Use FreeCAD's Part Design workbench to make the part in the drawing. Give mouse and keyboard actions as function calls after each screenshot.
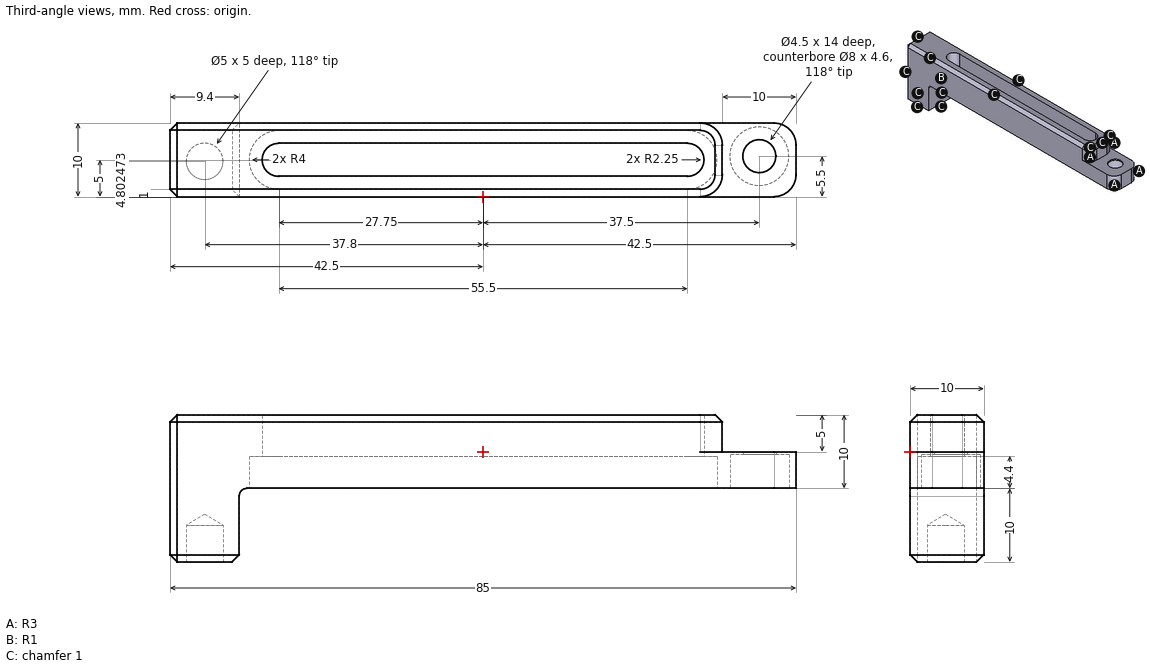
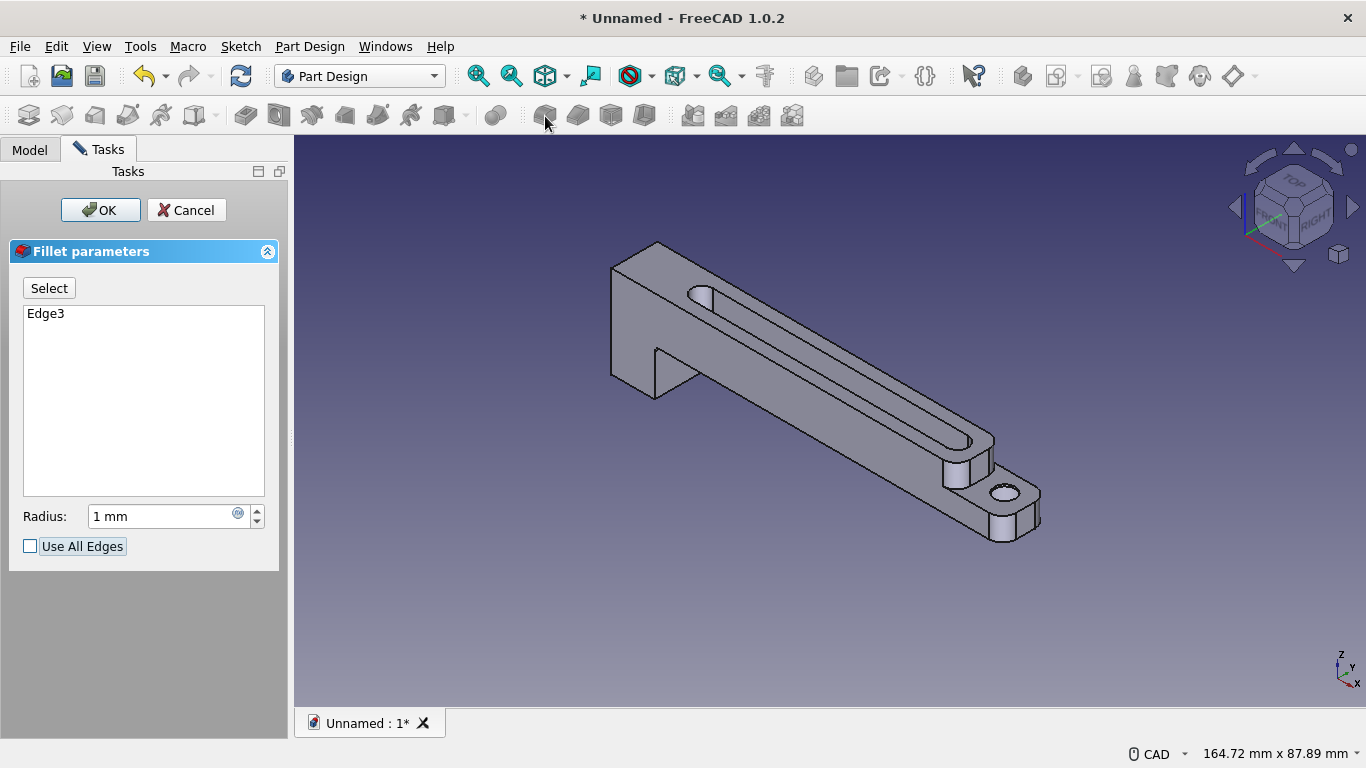
click(101, 210)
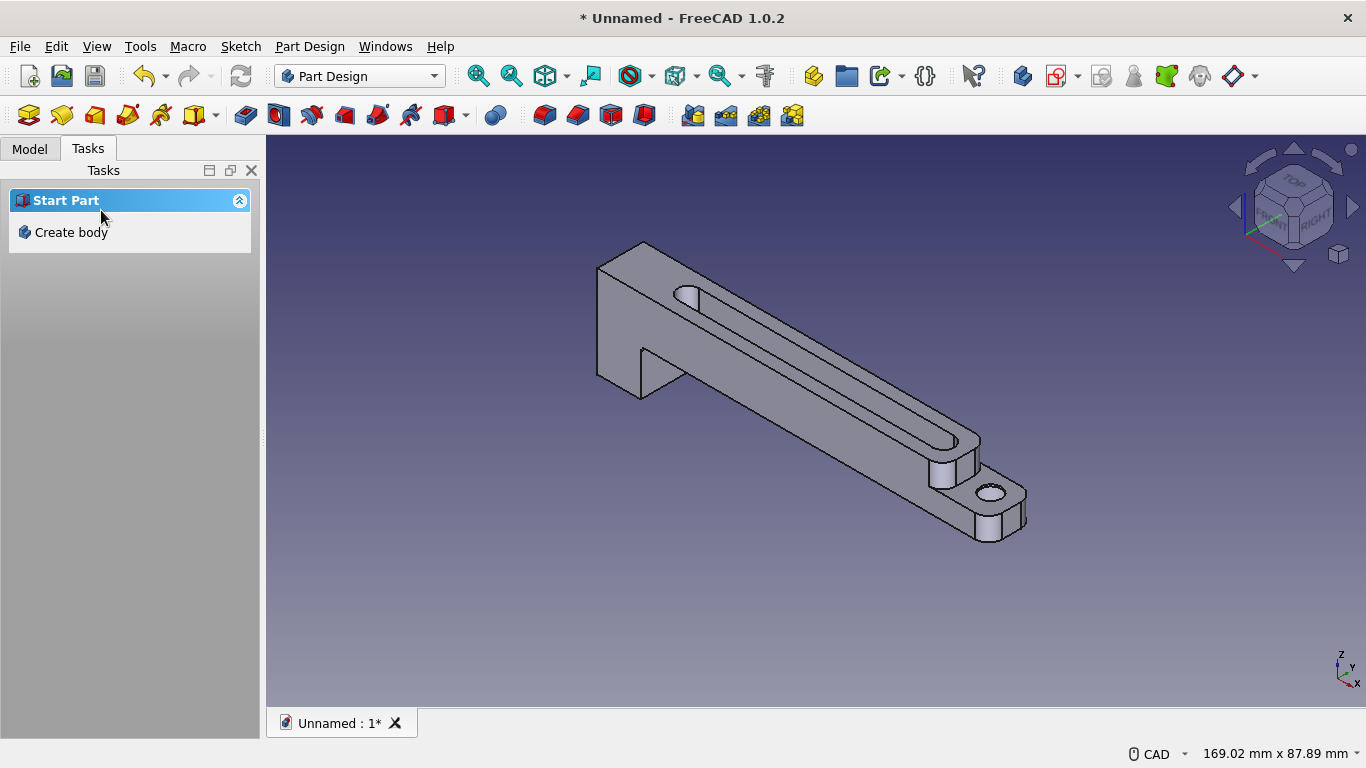
click(763, 363)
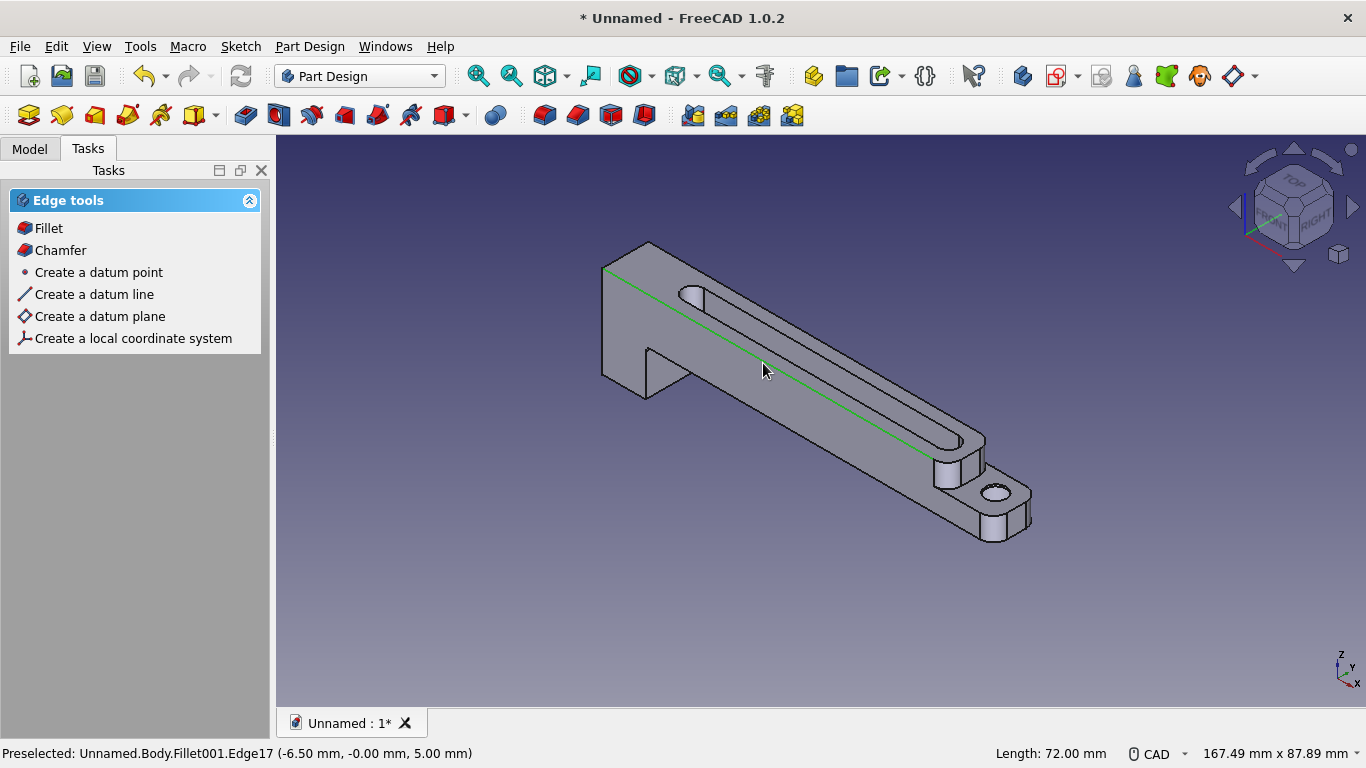
click(971, 453, ctrl)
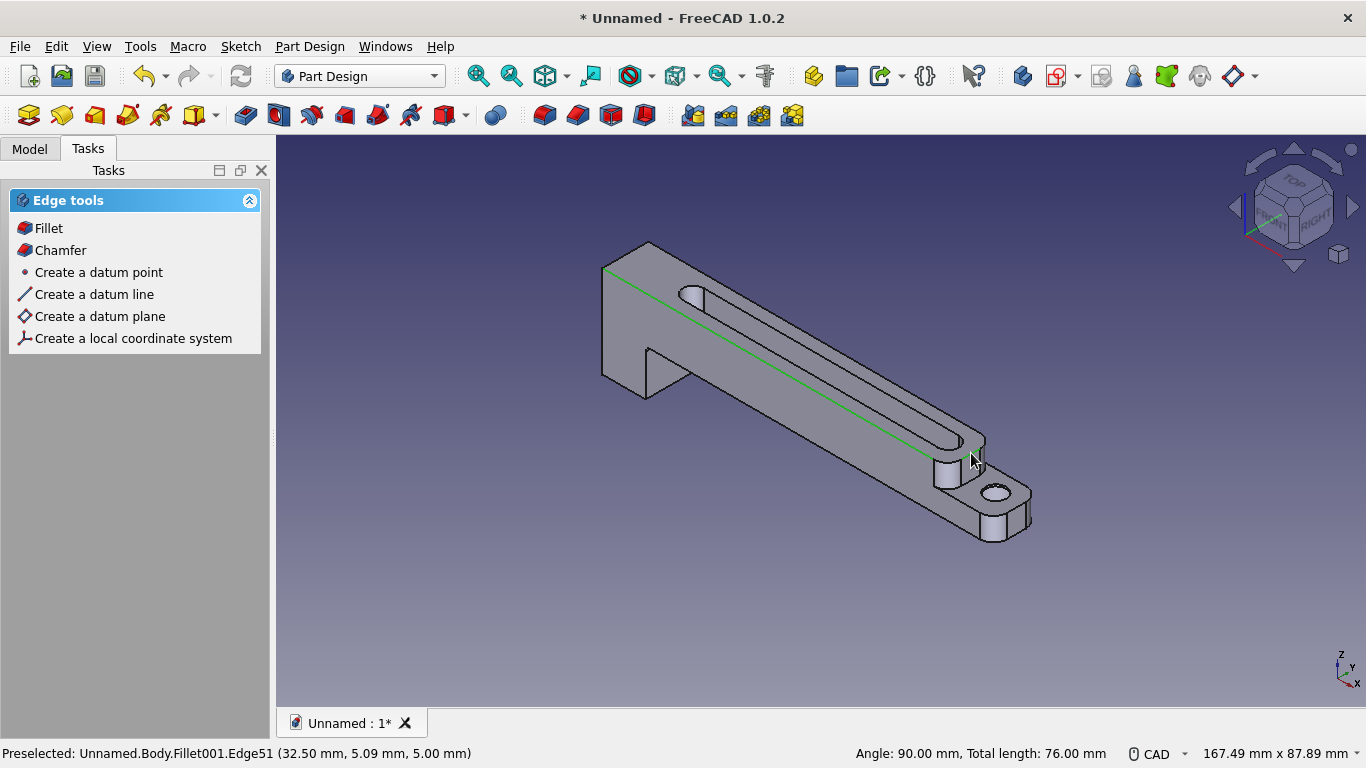
click(985, 440, ctrl)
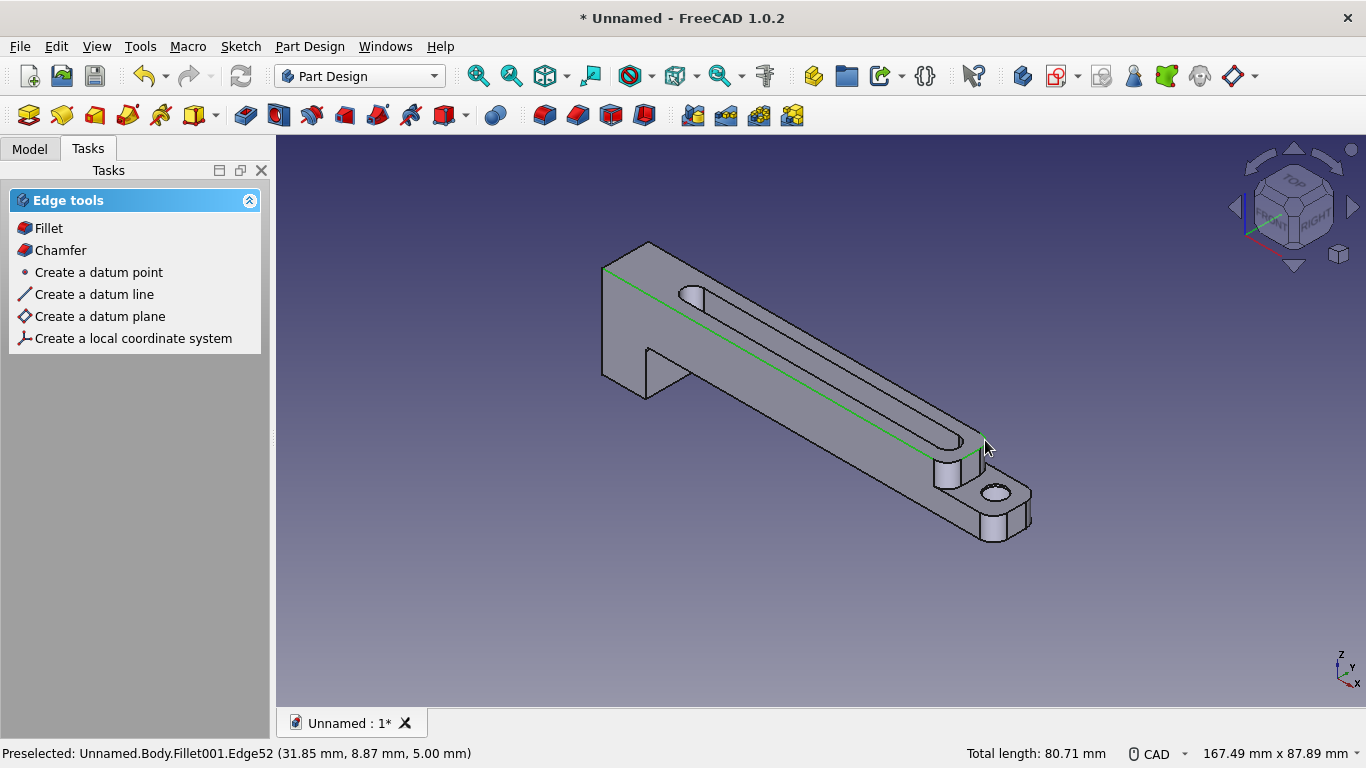
click(948, 462, ctrl)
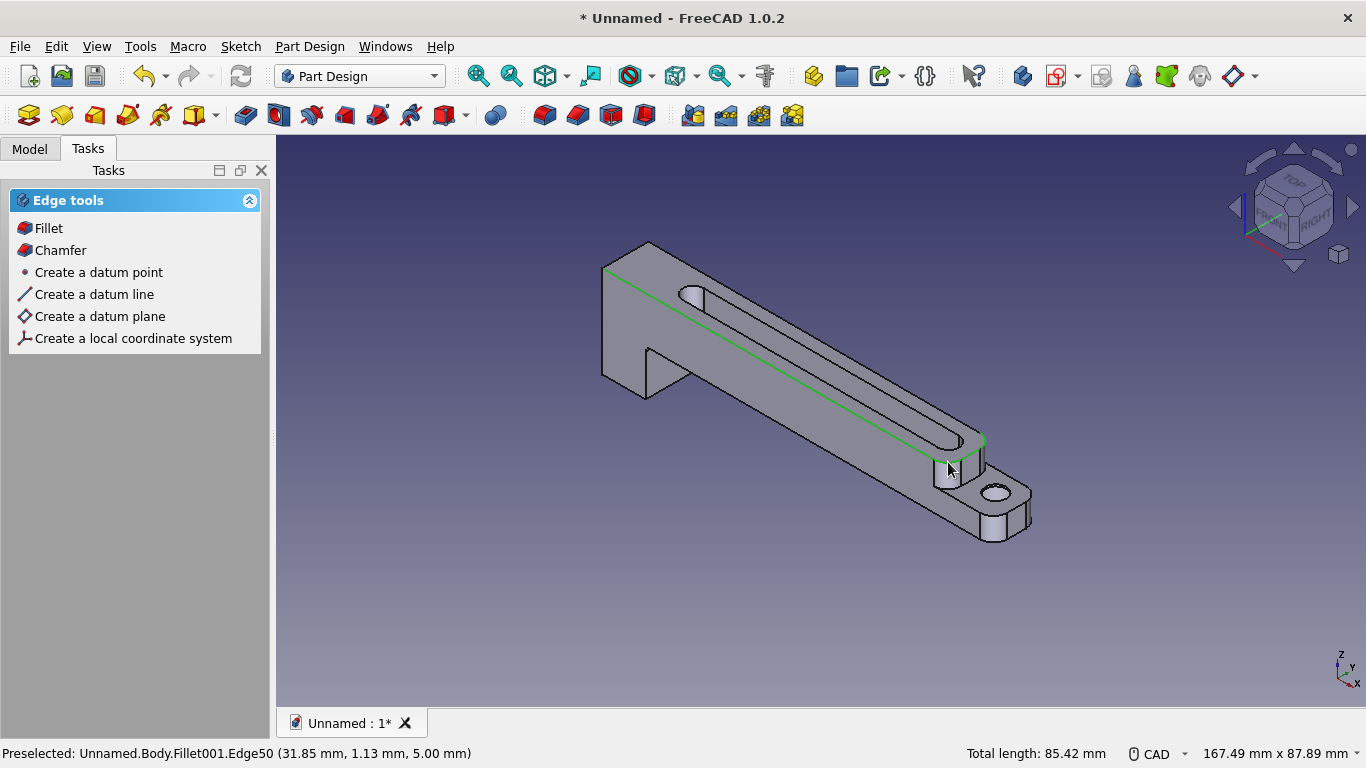
key(2)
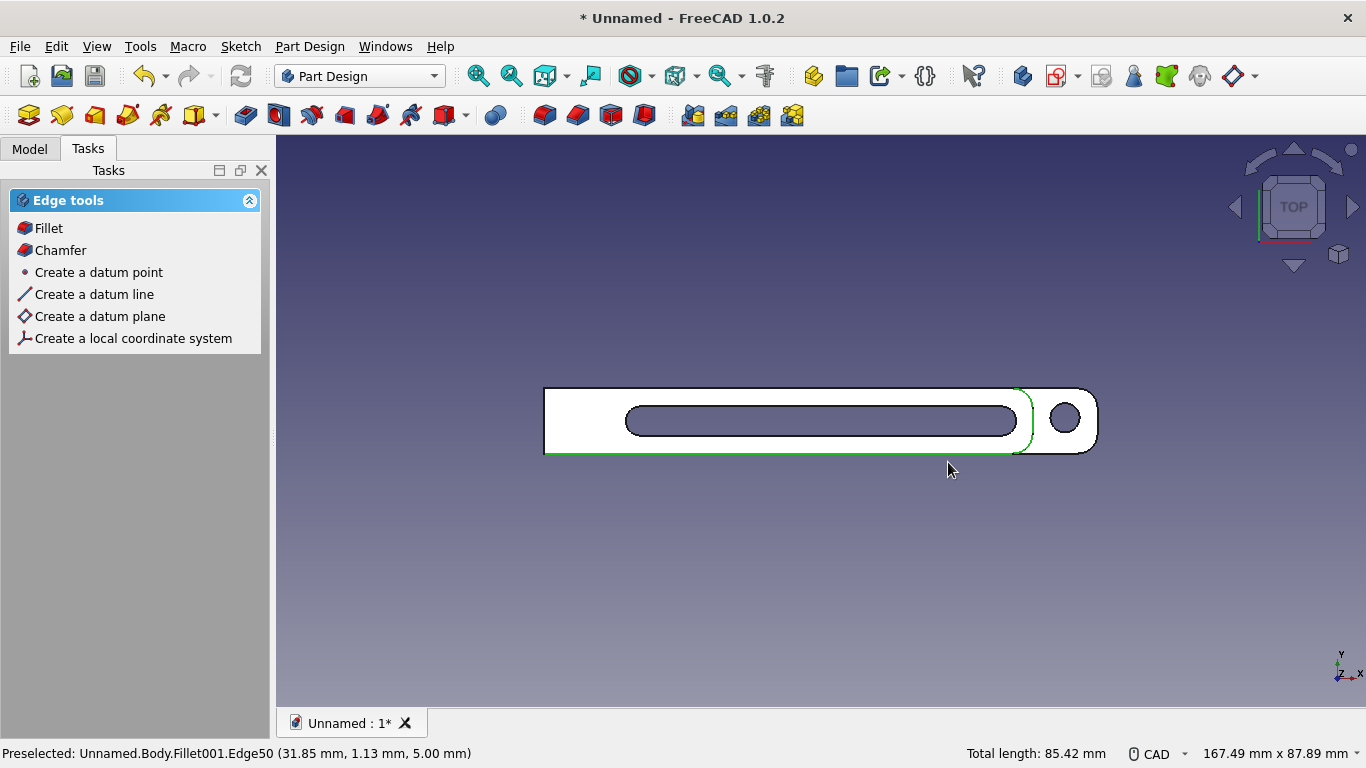
click(779, 387, ctrl)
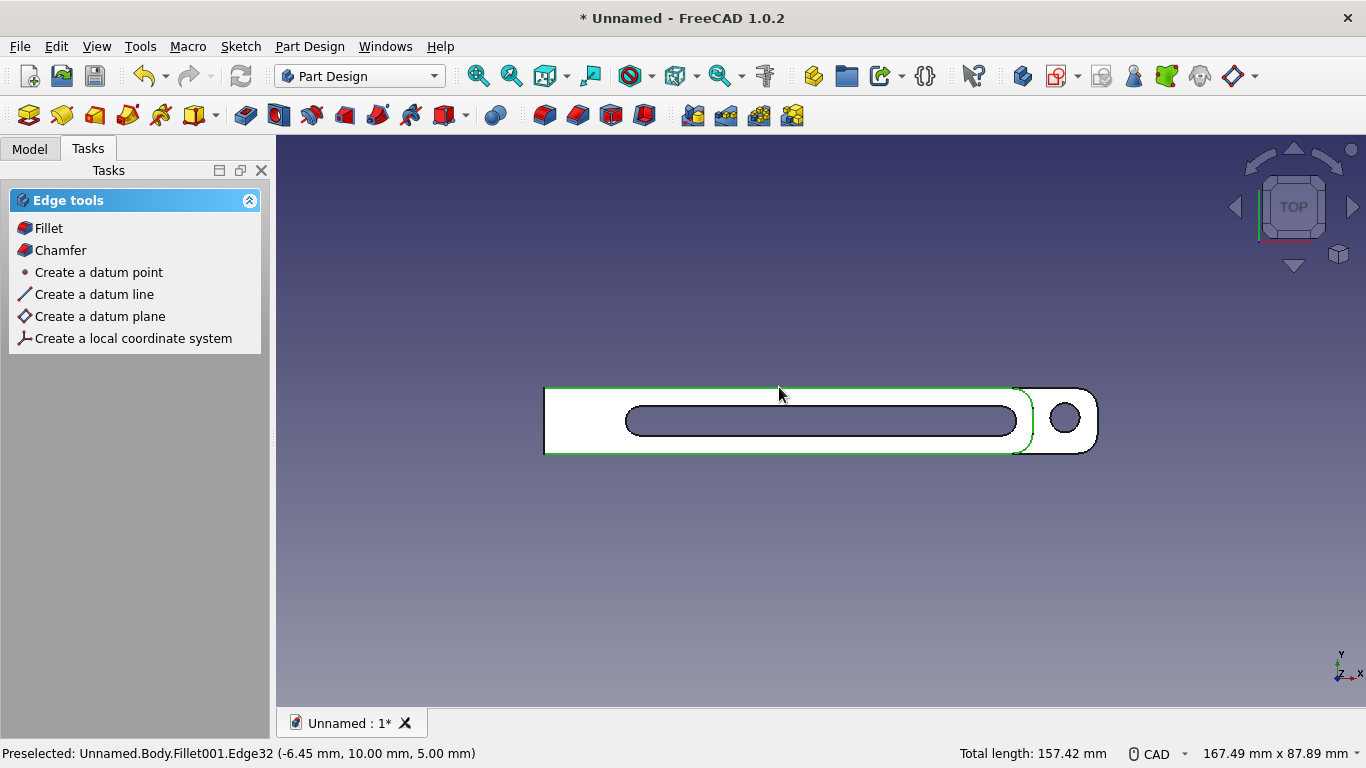
key(0)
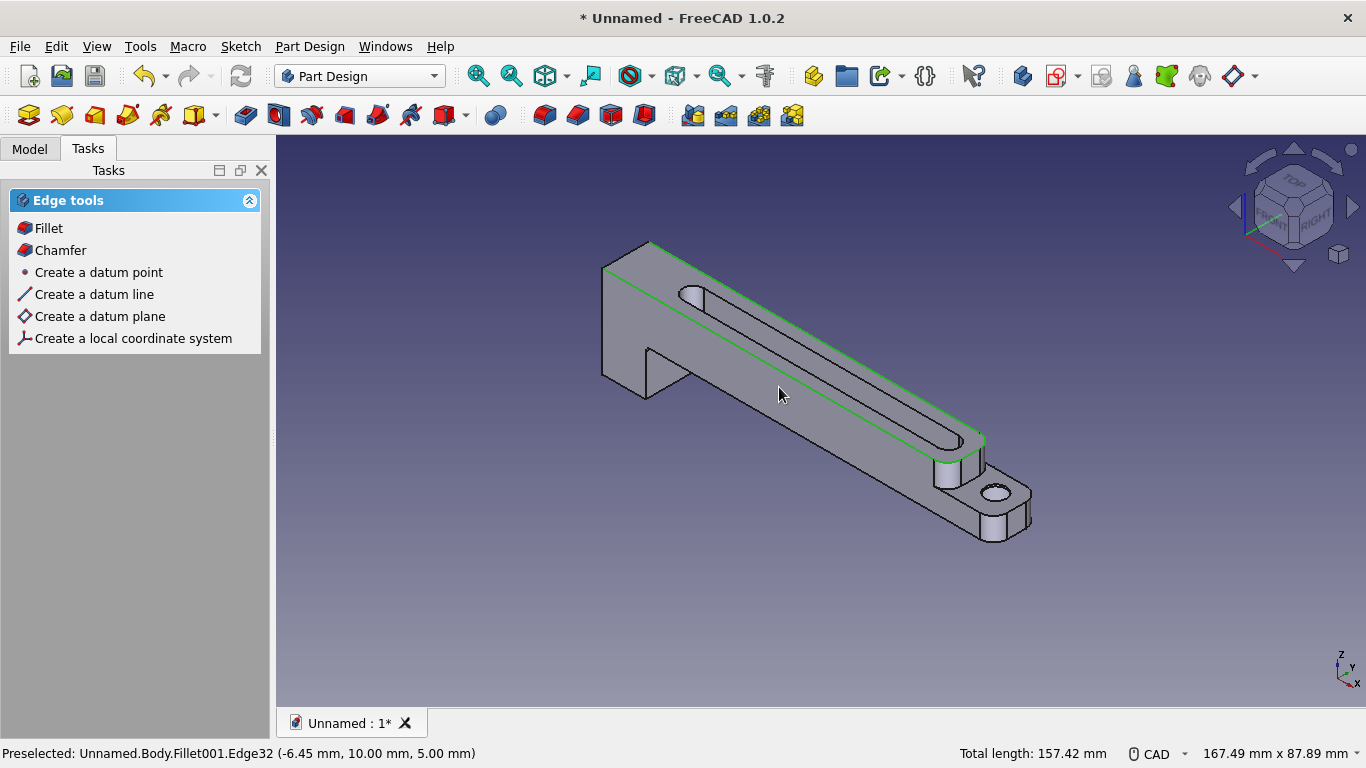
key(1)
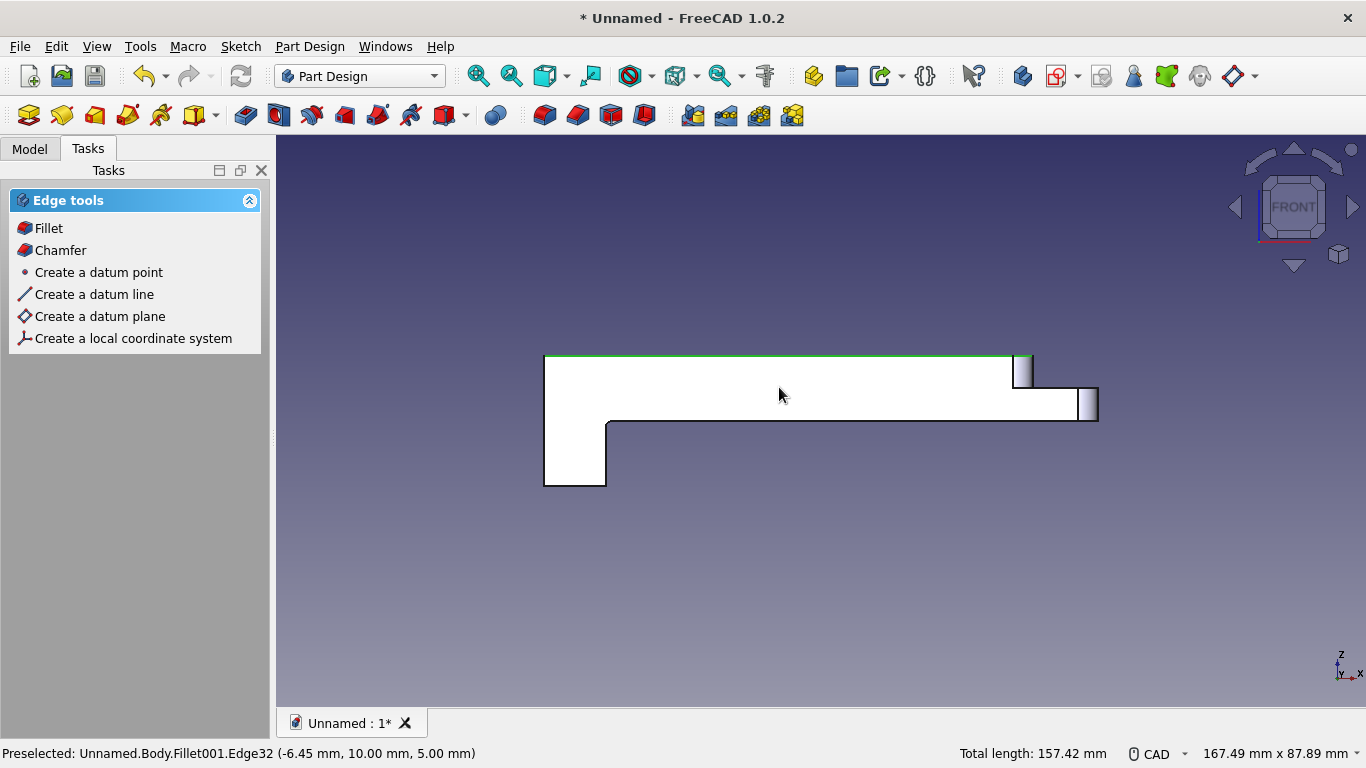
key(3)